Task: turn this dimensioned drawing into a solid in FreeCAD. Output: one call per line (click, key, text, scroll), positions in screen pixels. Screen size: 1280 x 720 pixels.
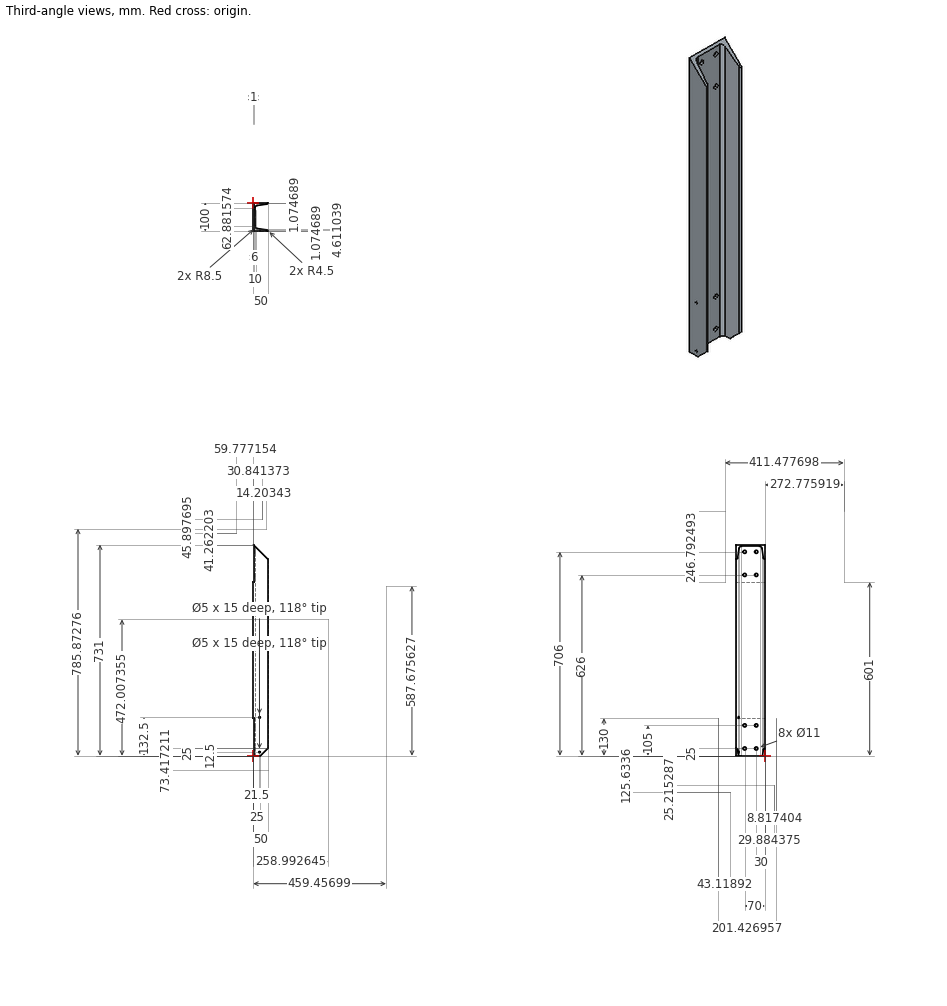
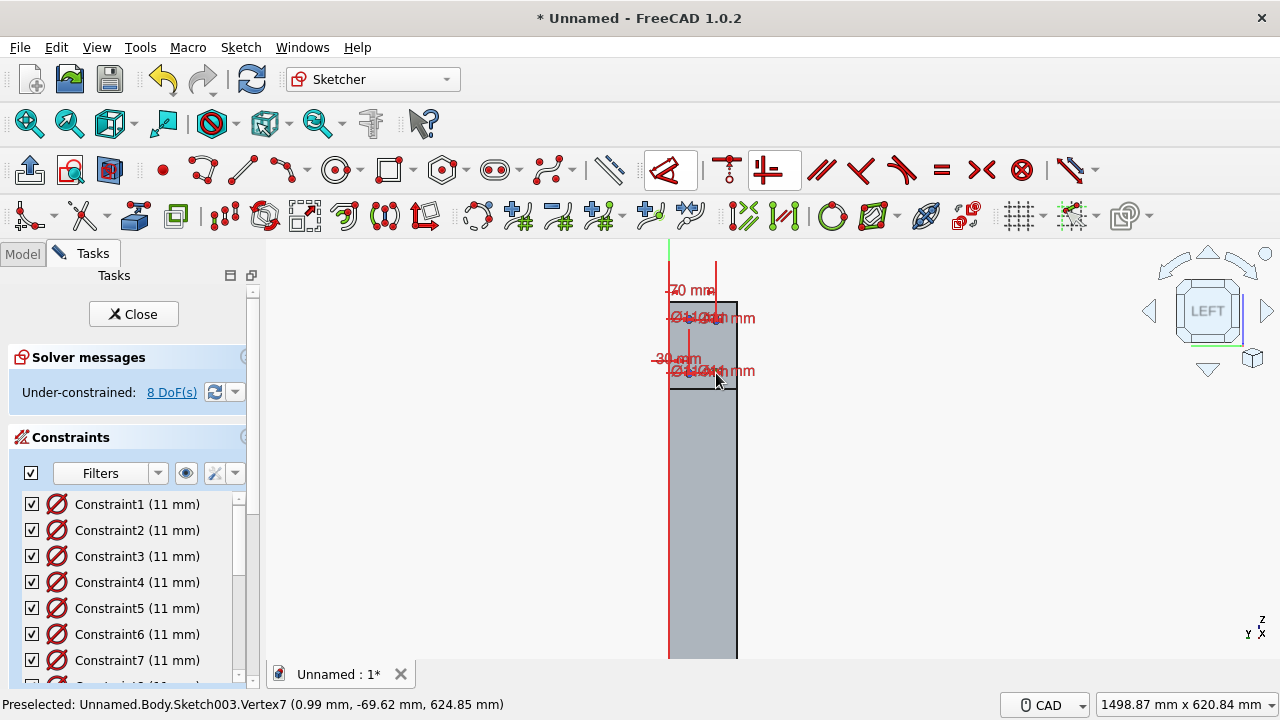
key(l)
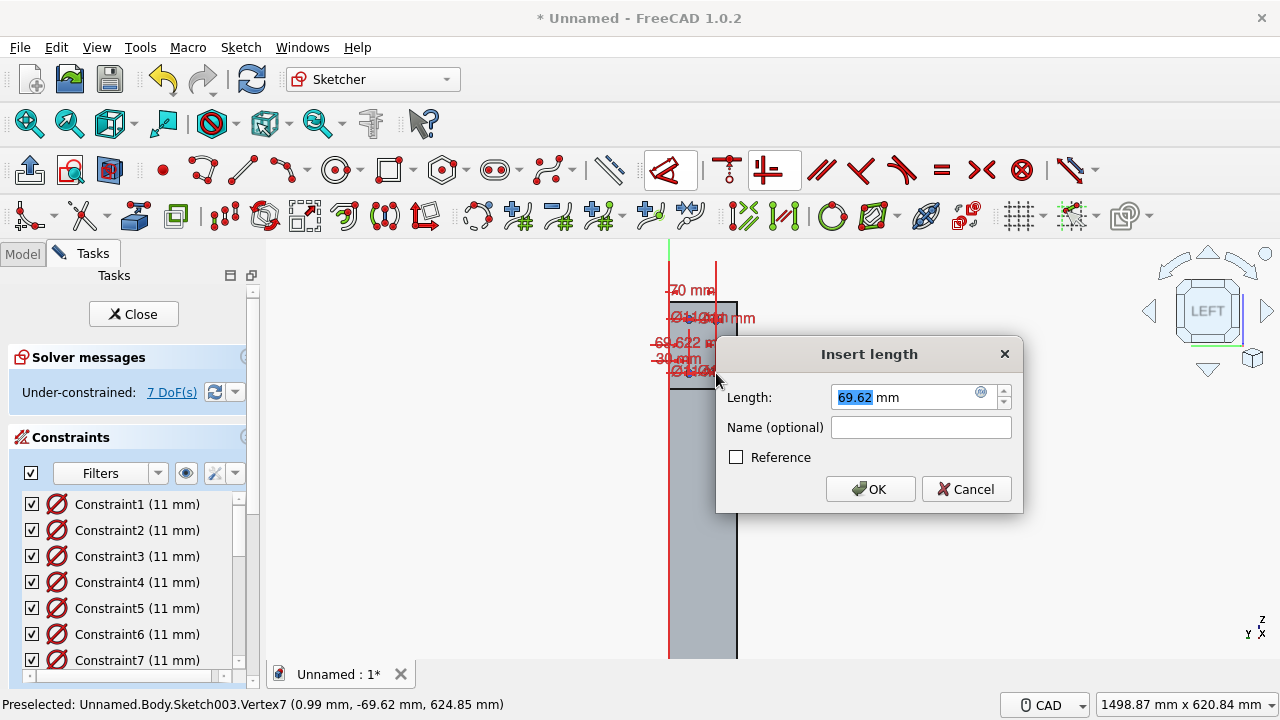
text(70)
key(Return)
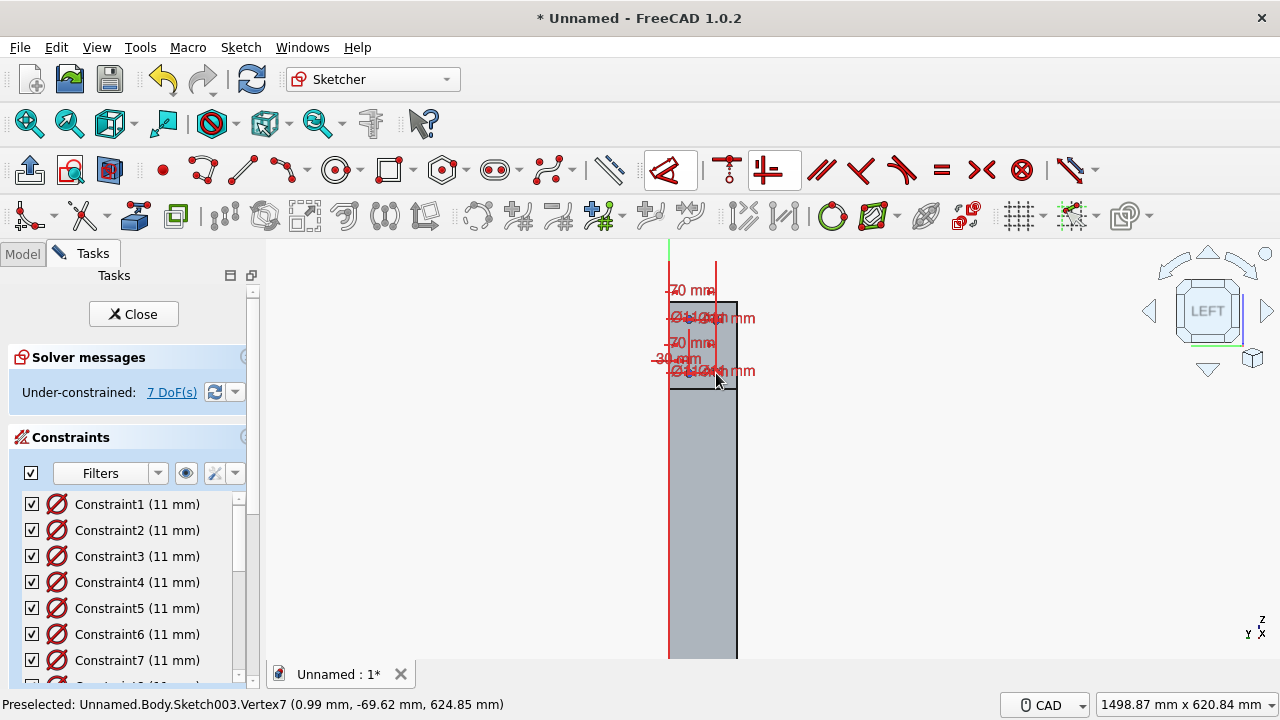
scroll(689, 319, up, 4)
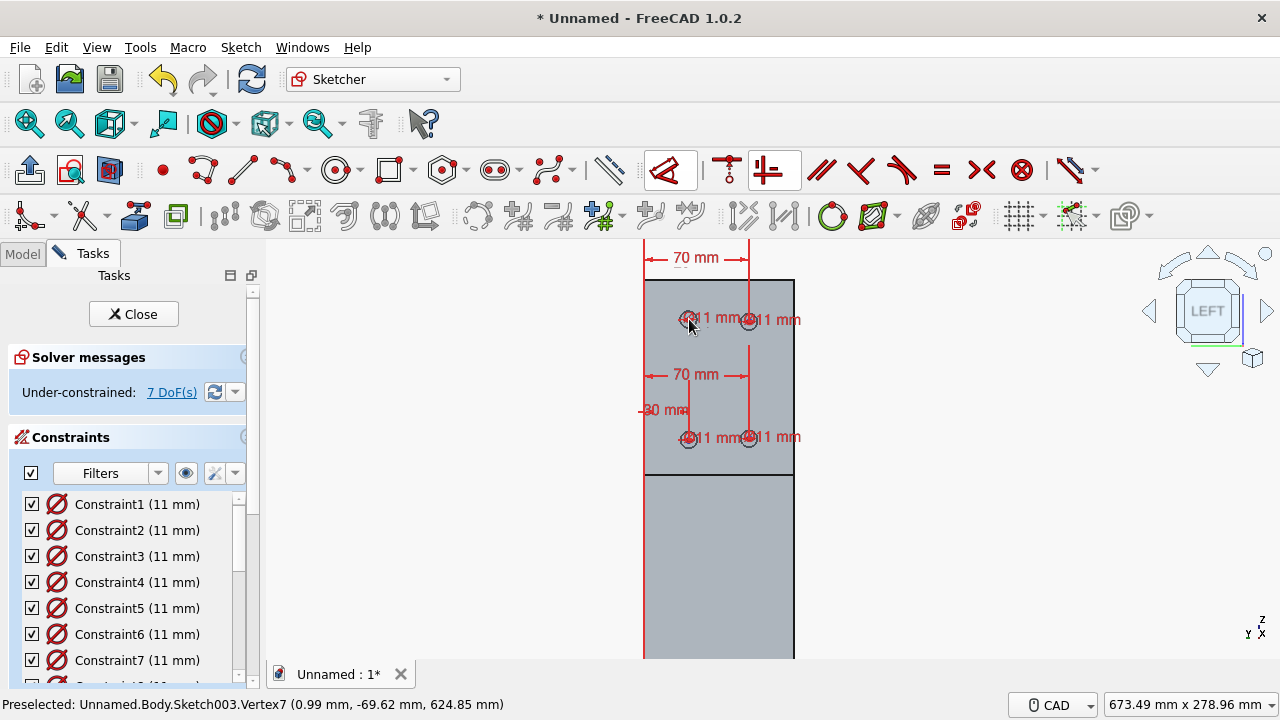
click(688, 320)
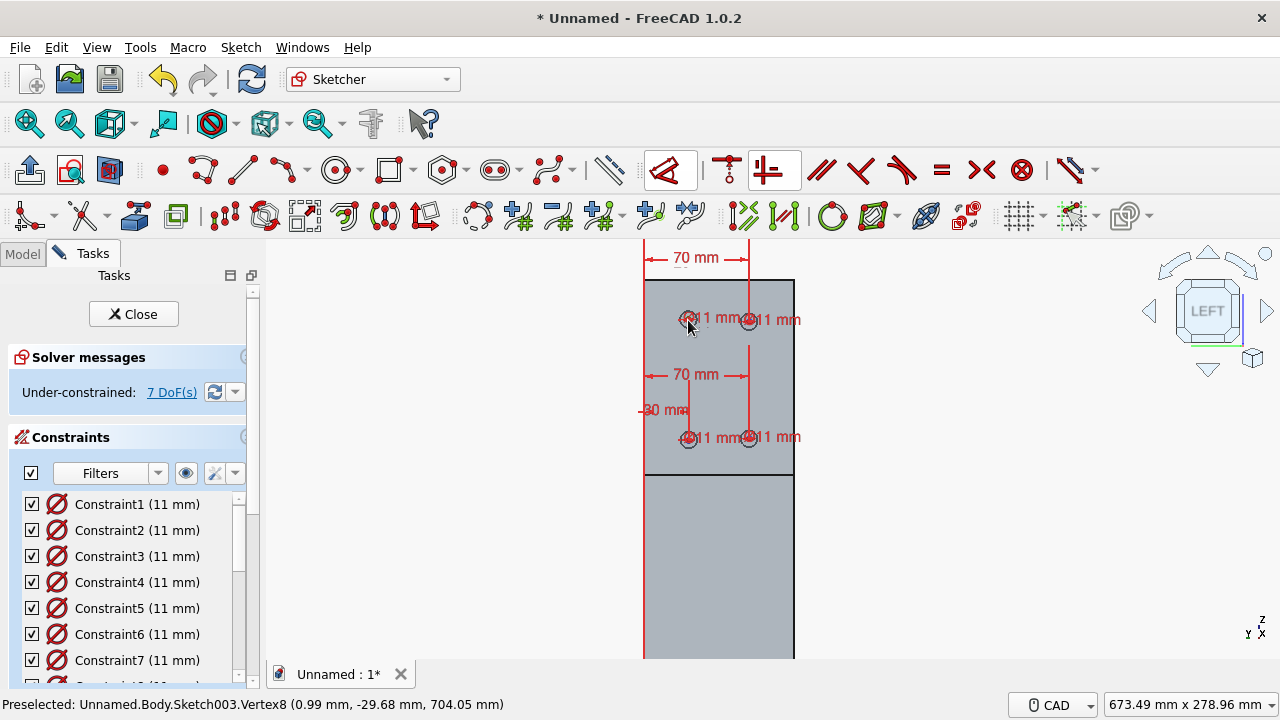
click(692, 170)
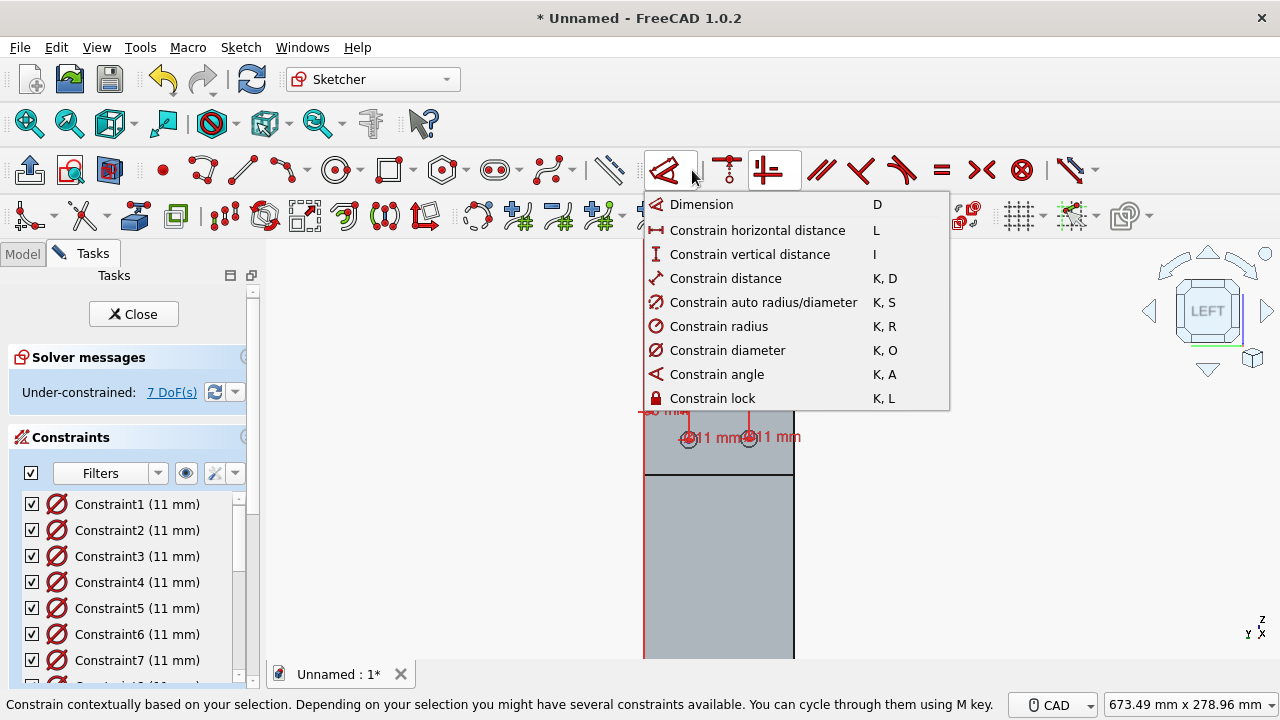
click(797, 230)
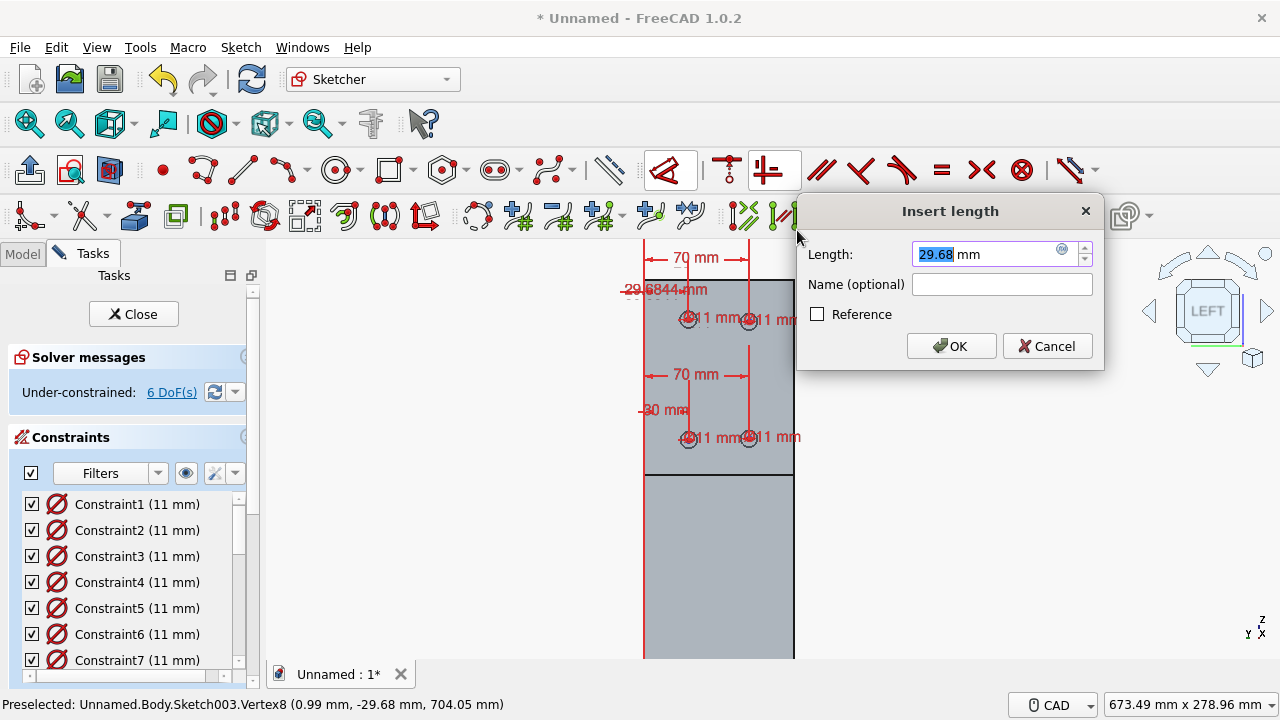
text(30)
key(Return)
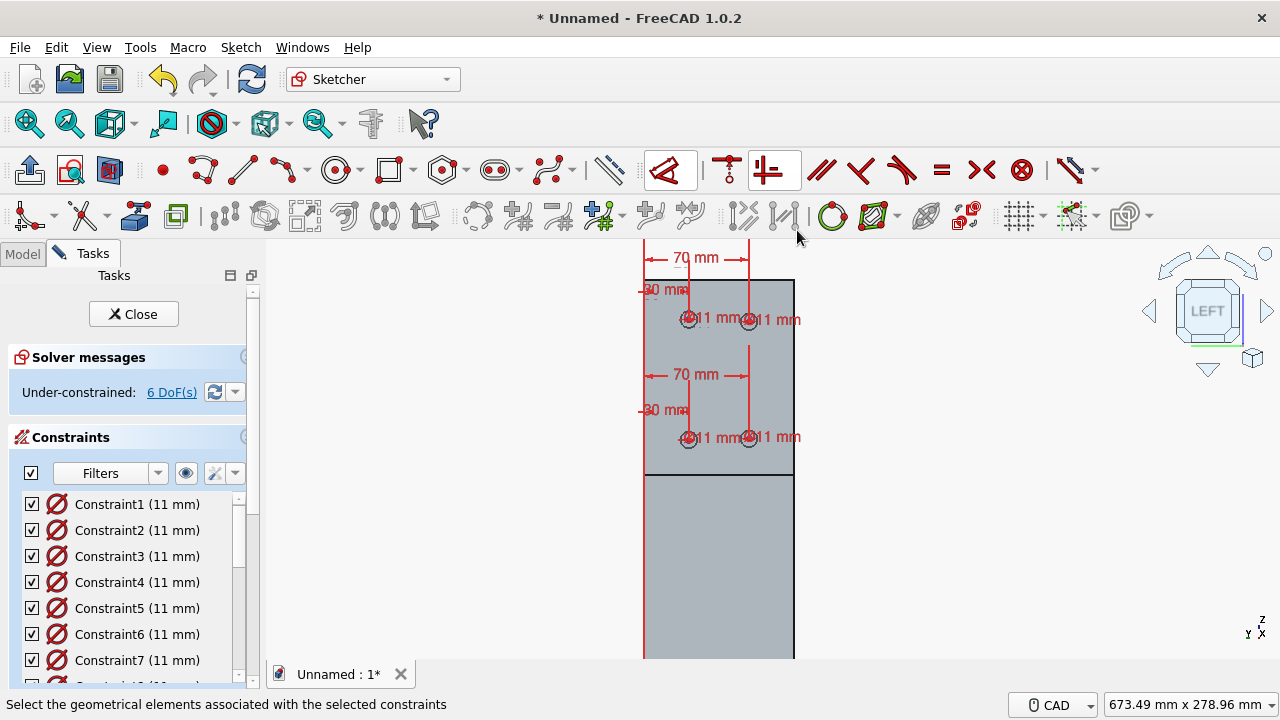
scroll(706, 320, down, 7)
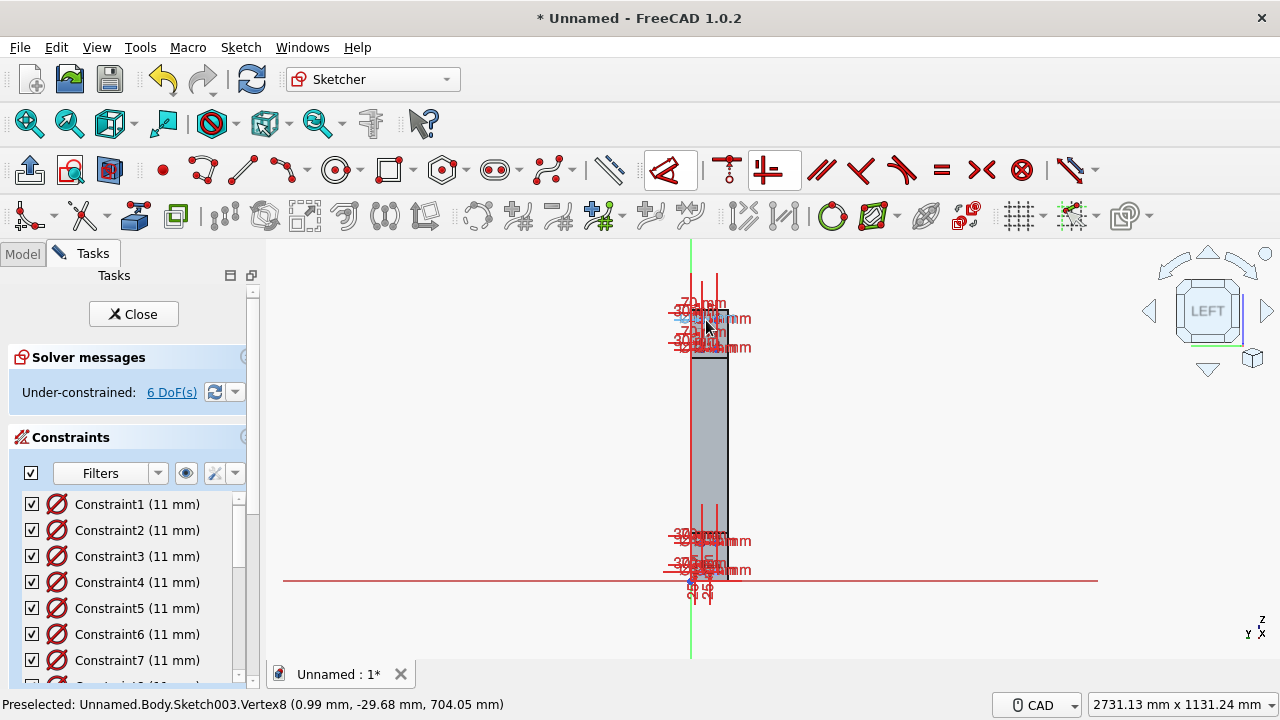
click(702, 543)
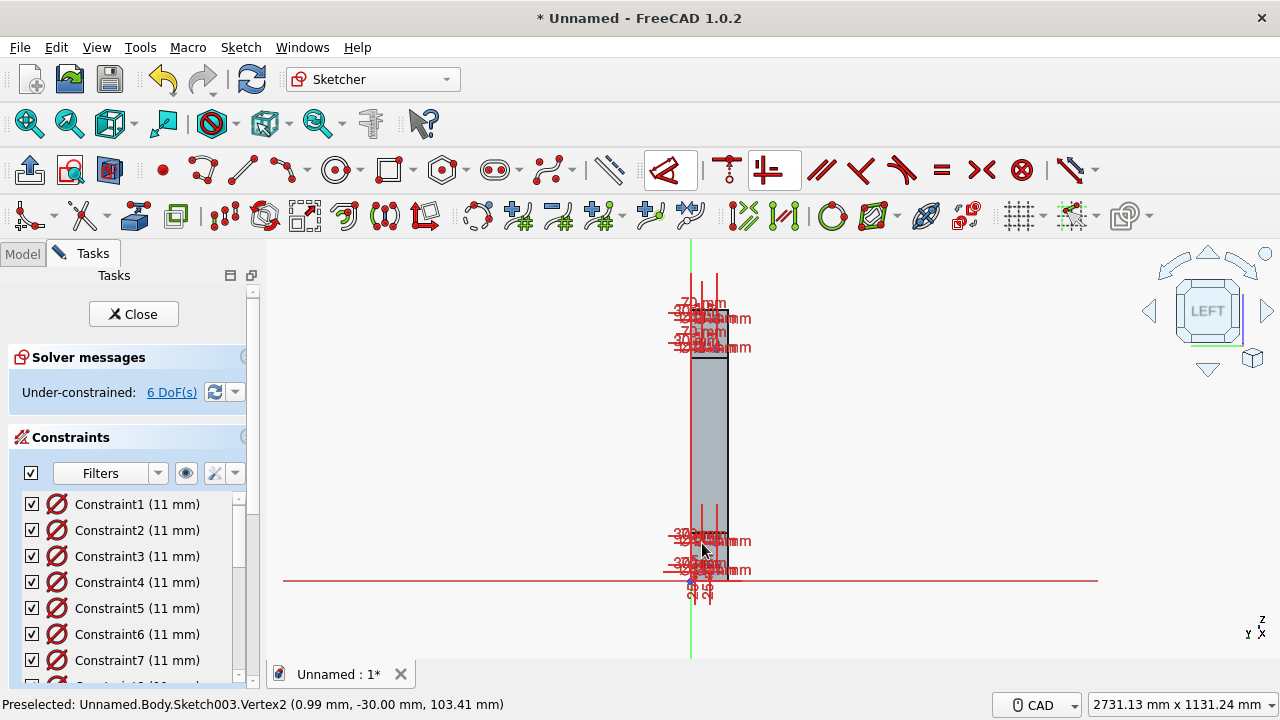
key(i)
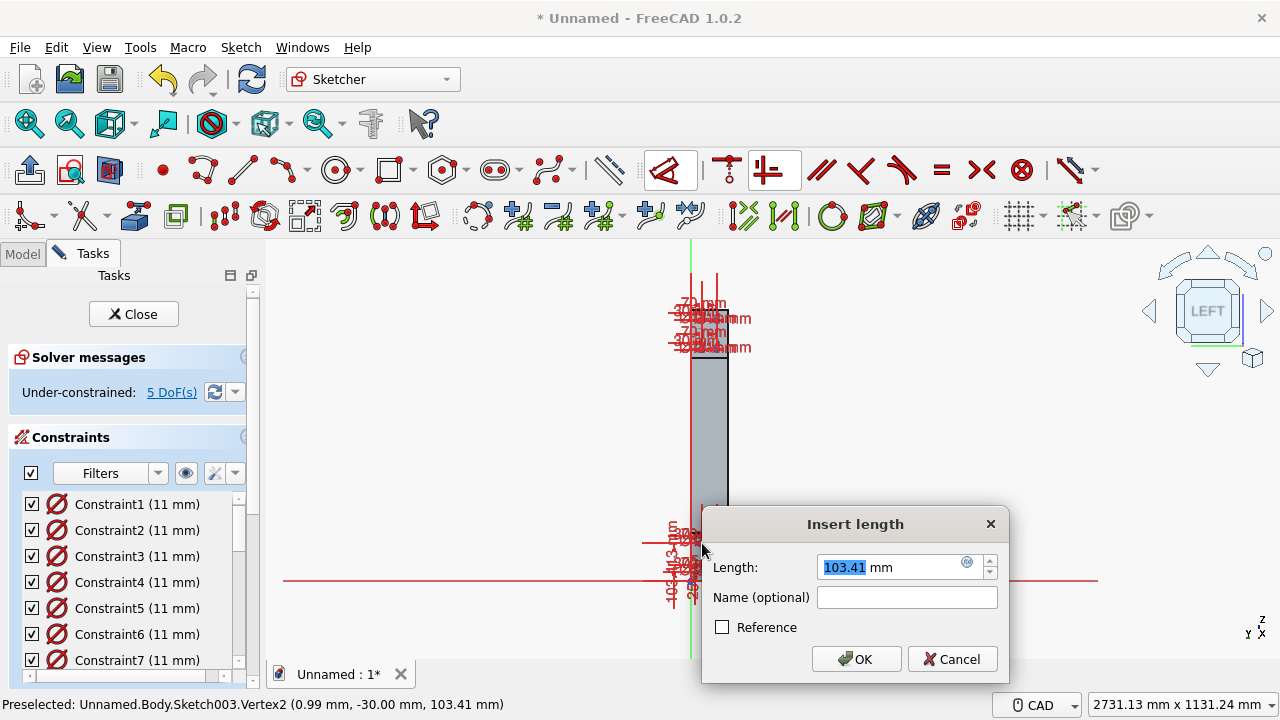
text(105)
key(Return)